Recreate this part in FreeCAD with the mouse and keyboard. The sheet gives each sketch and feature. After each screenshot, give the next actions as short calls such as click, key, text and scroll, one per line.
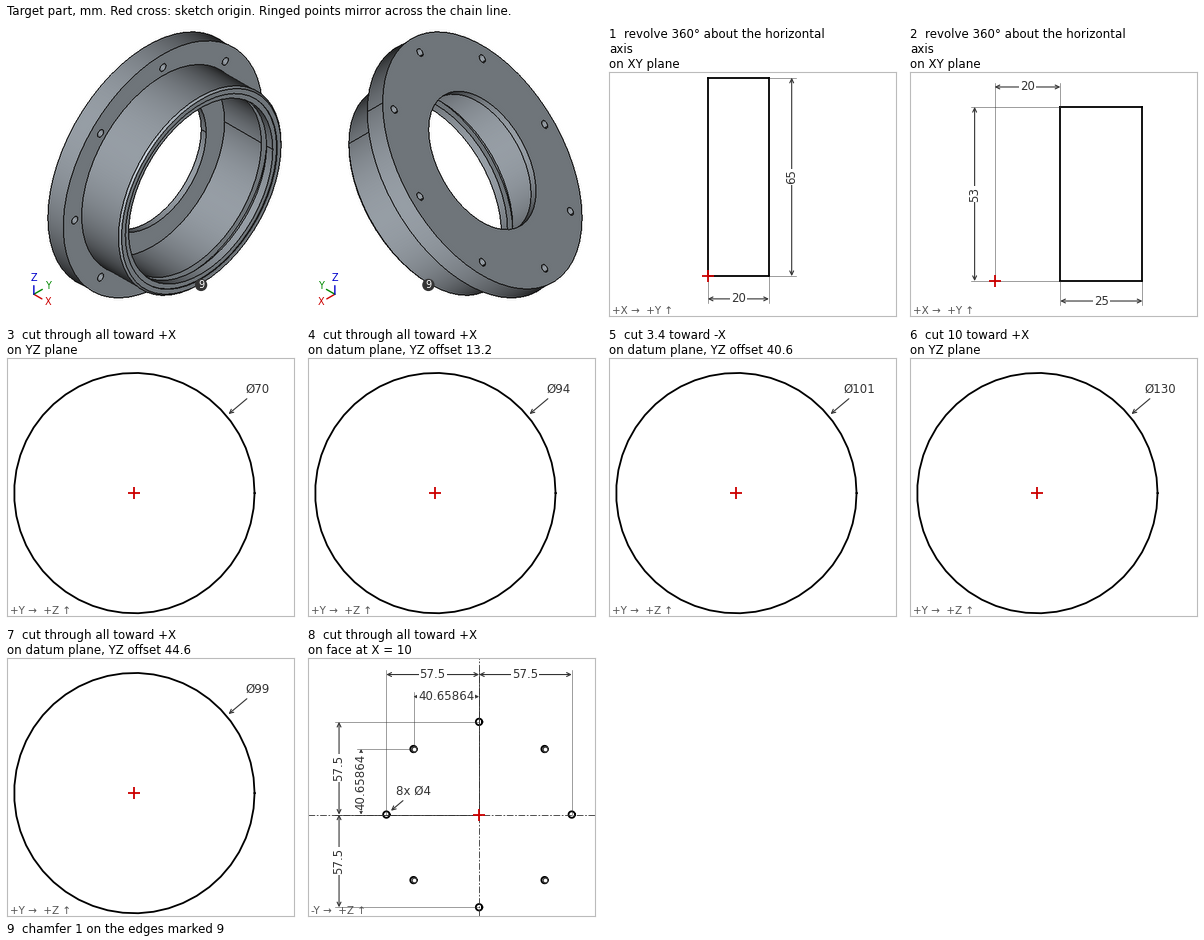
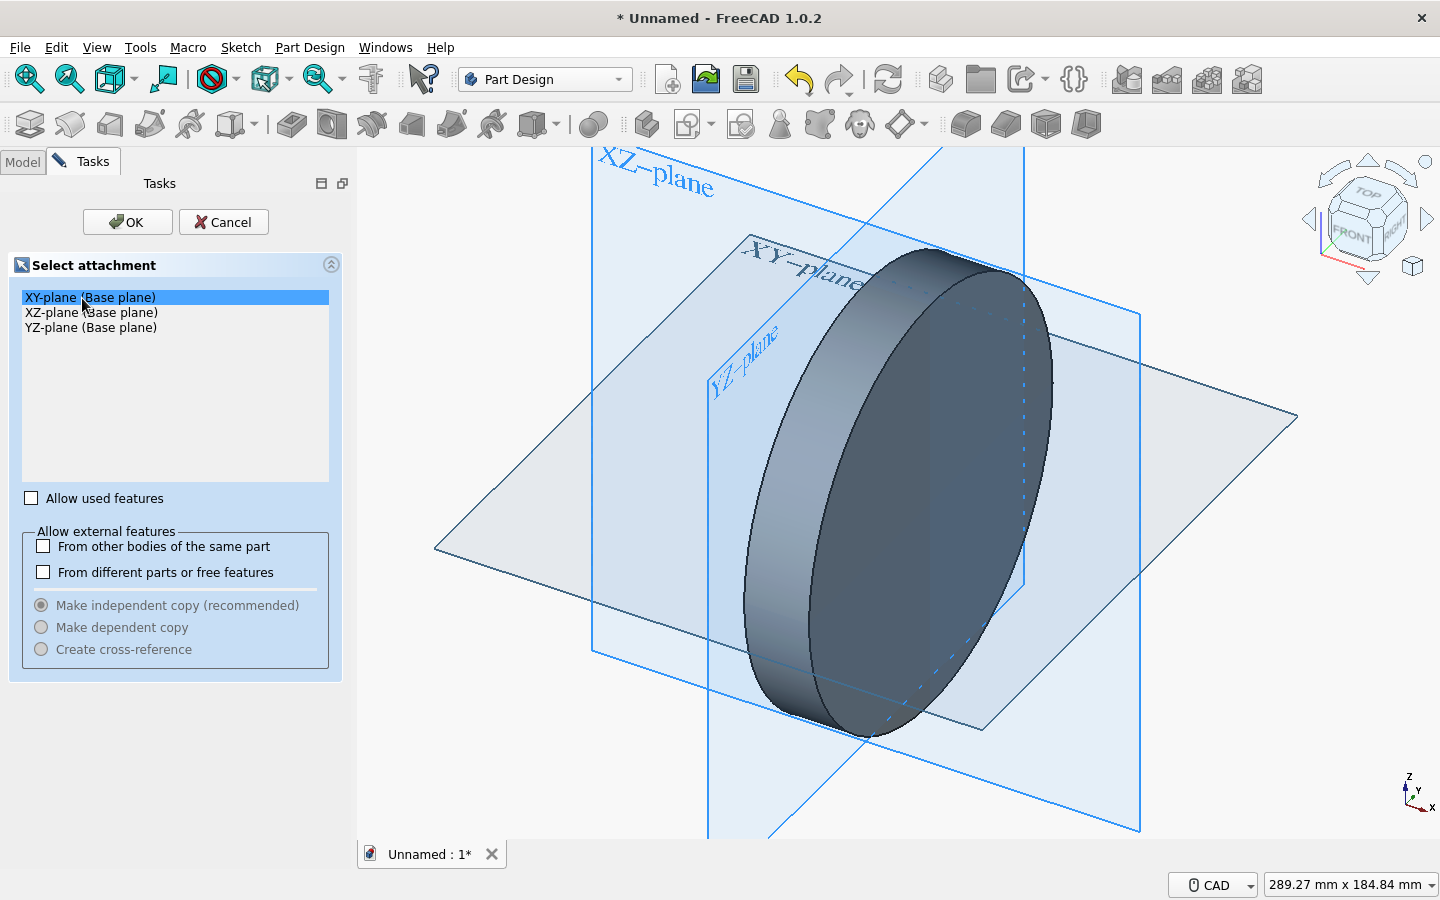
click(128, 222)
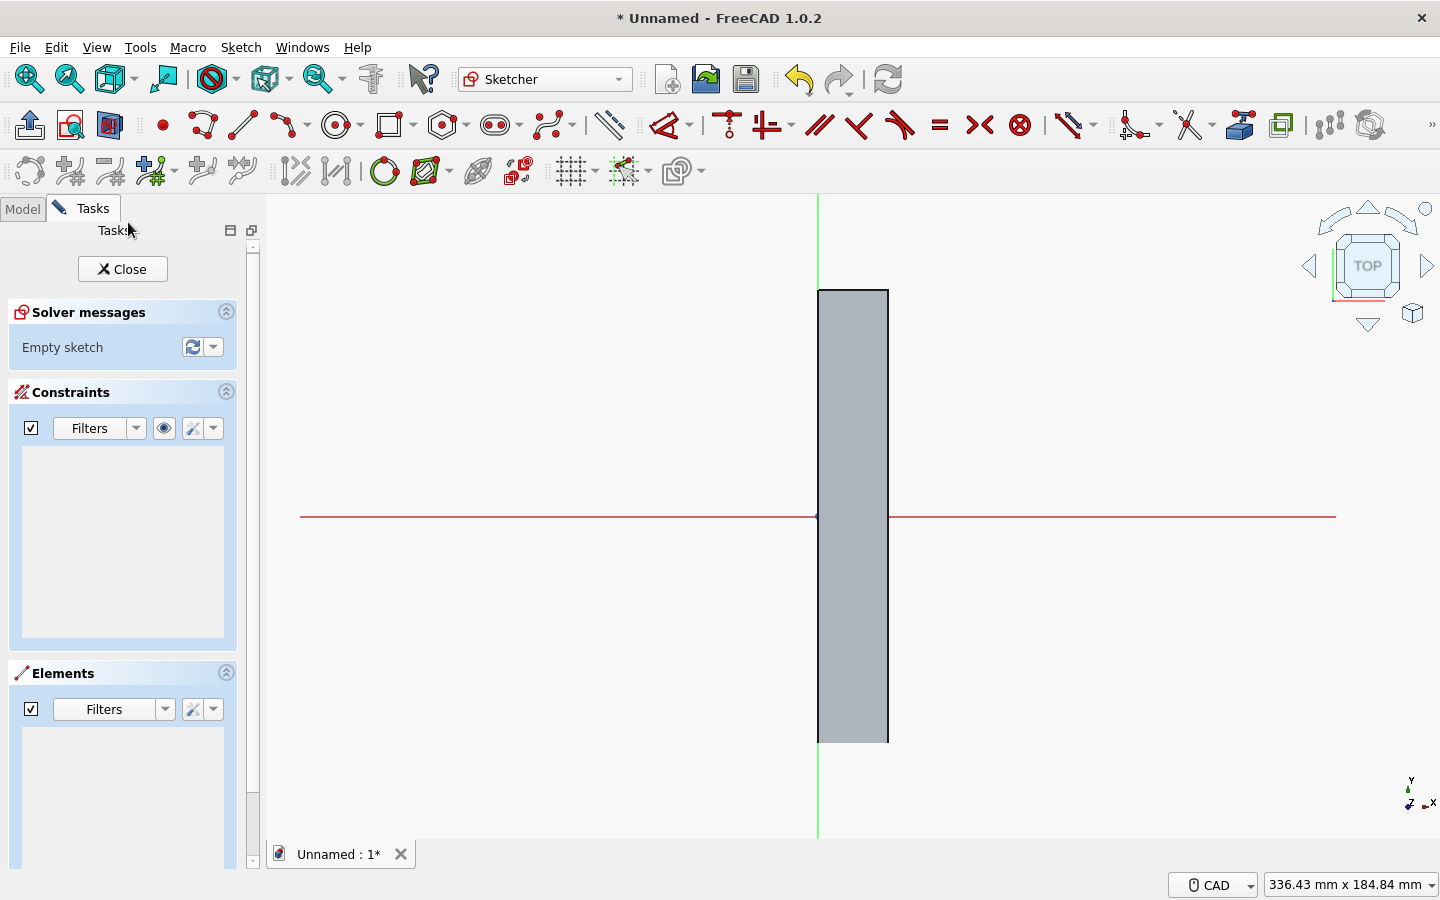
click(110, 126)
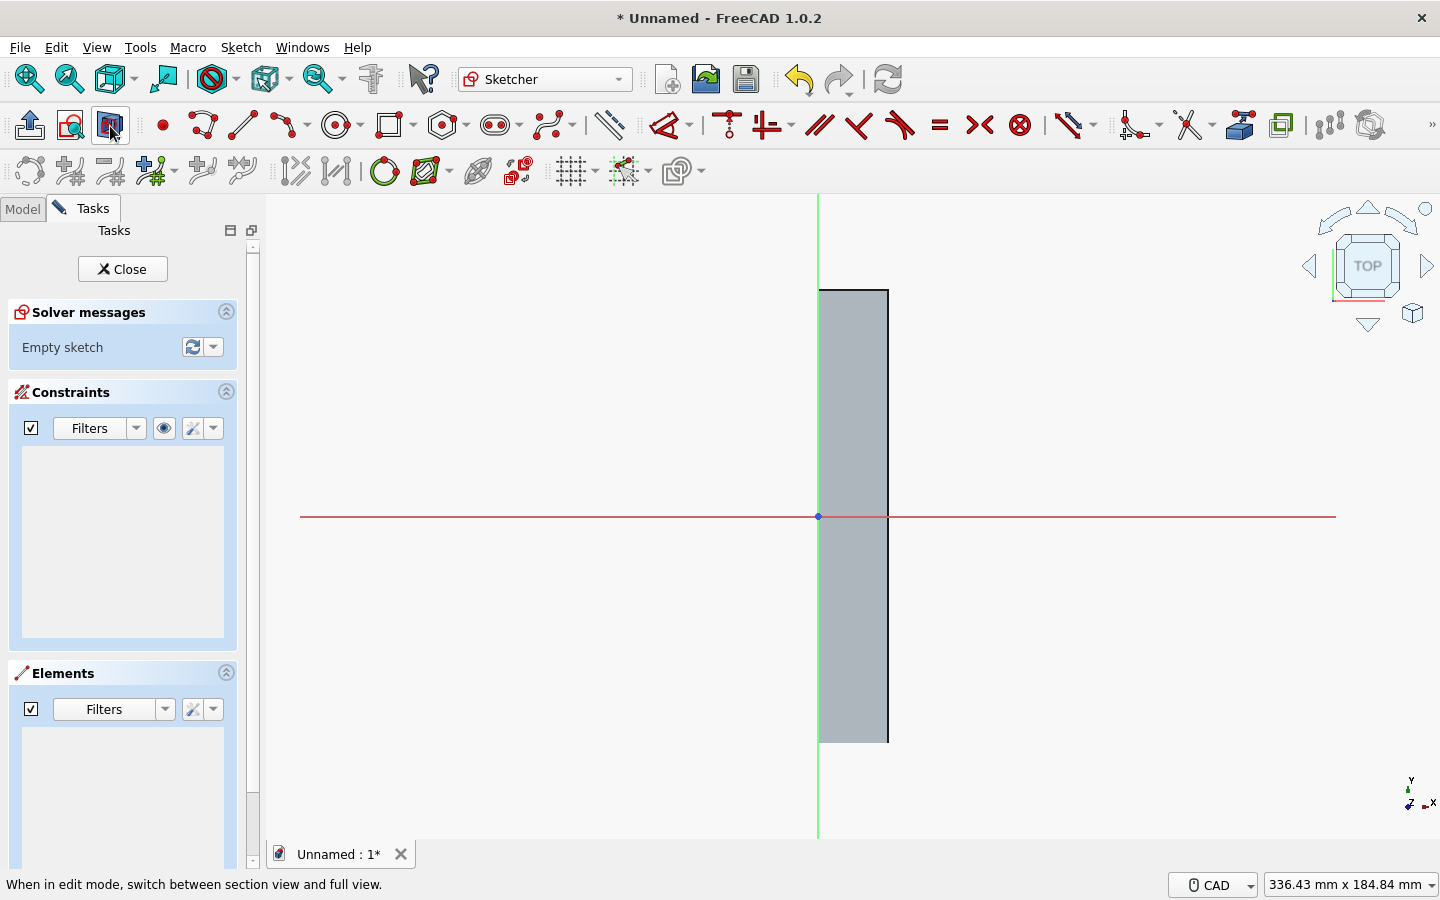
scroll(988, 349, up, 4)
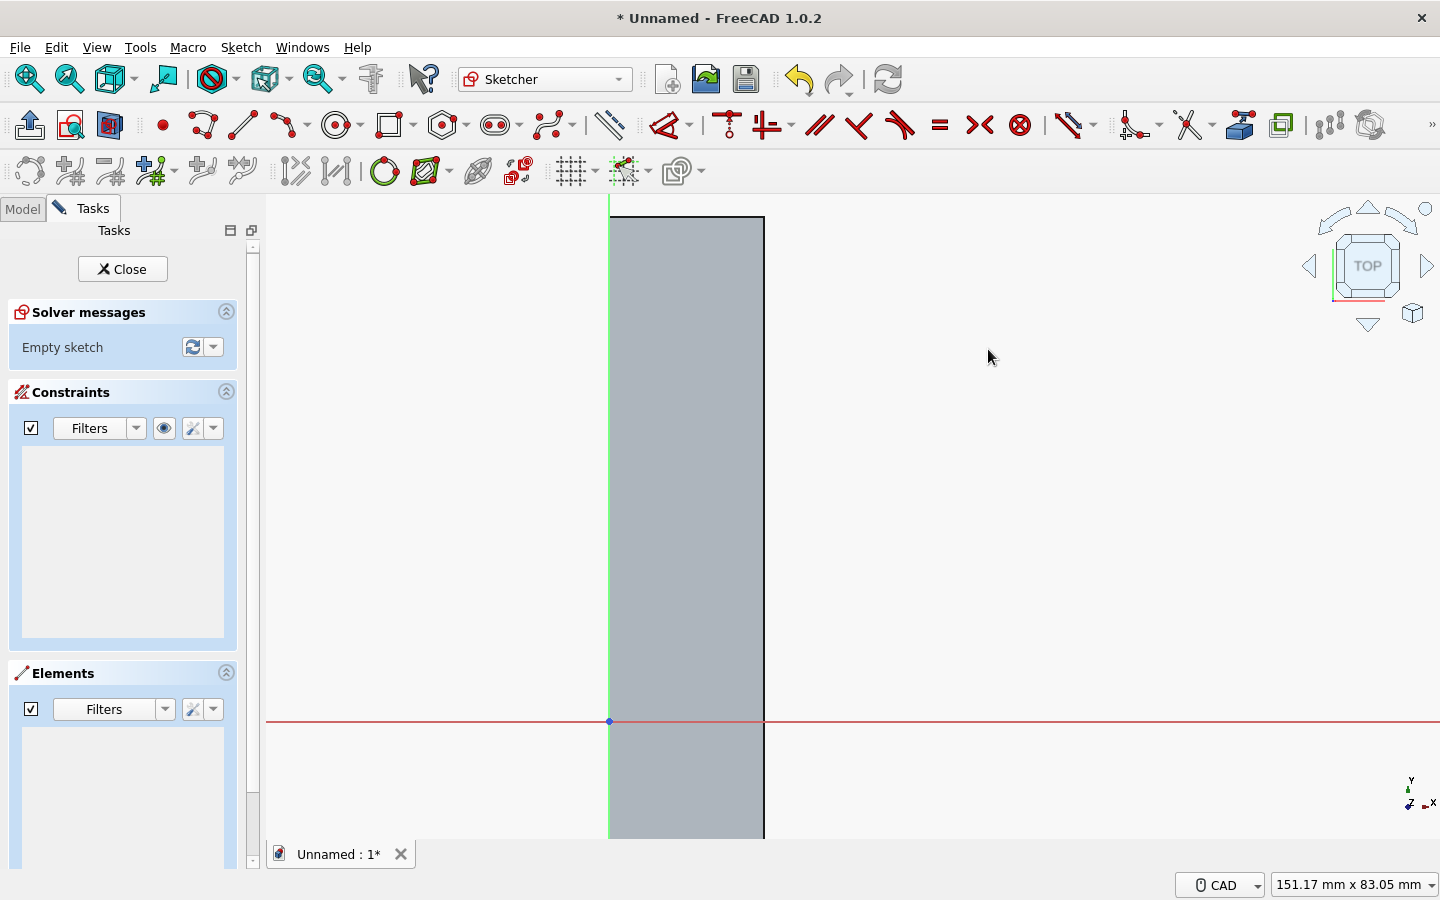
click(390, 126)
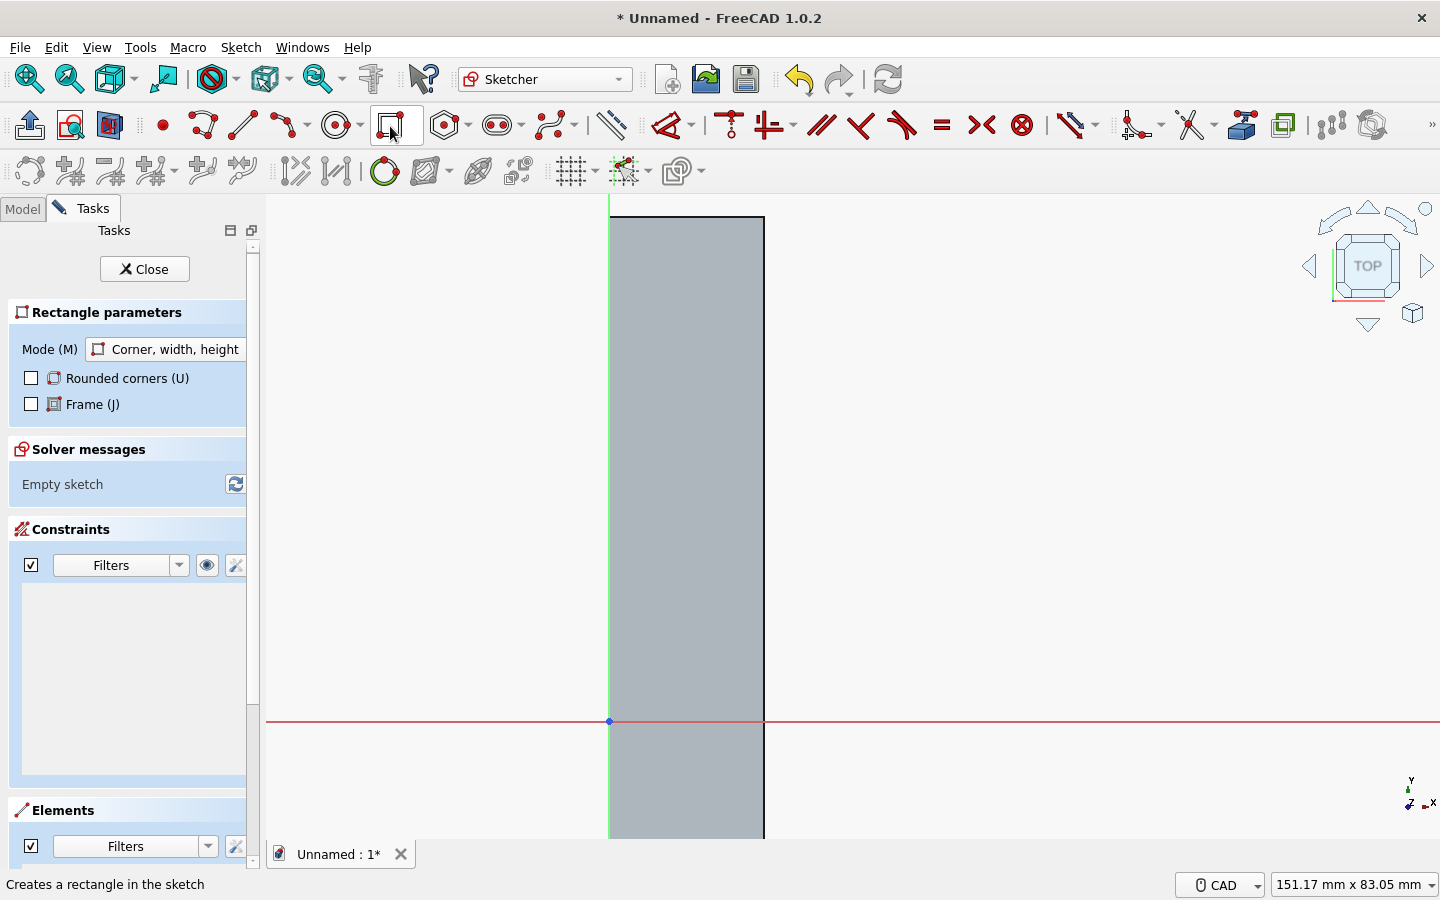
click(764, 310)
click(959, 722)
key(Escape)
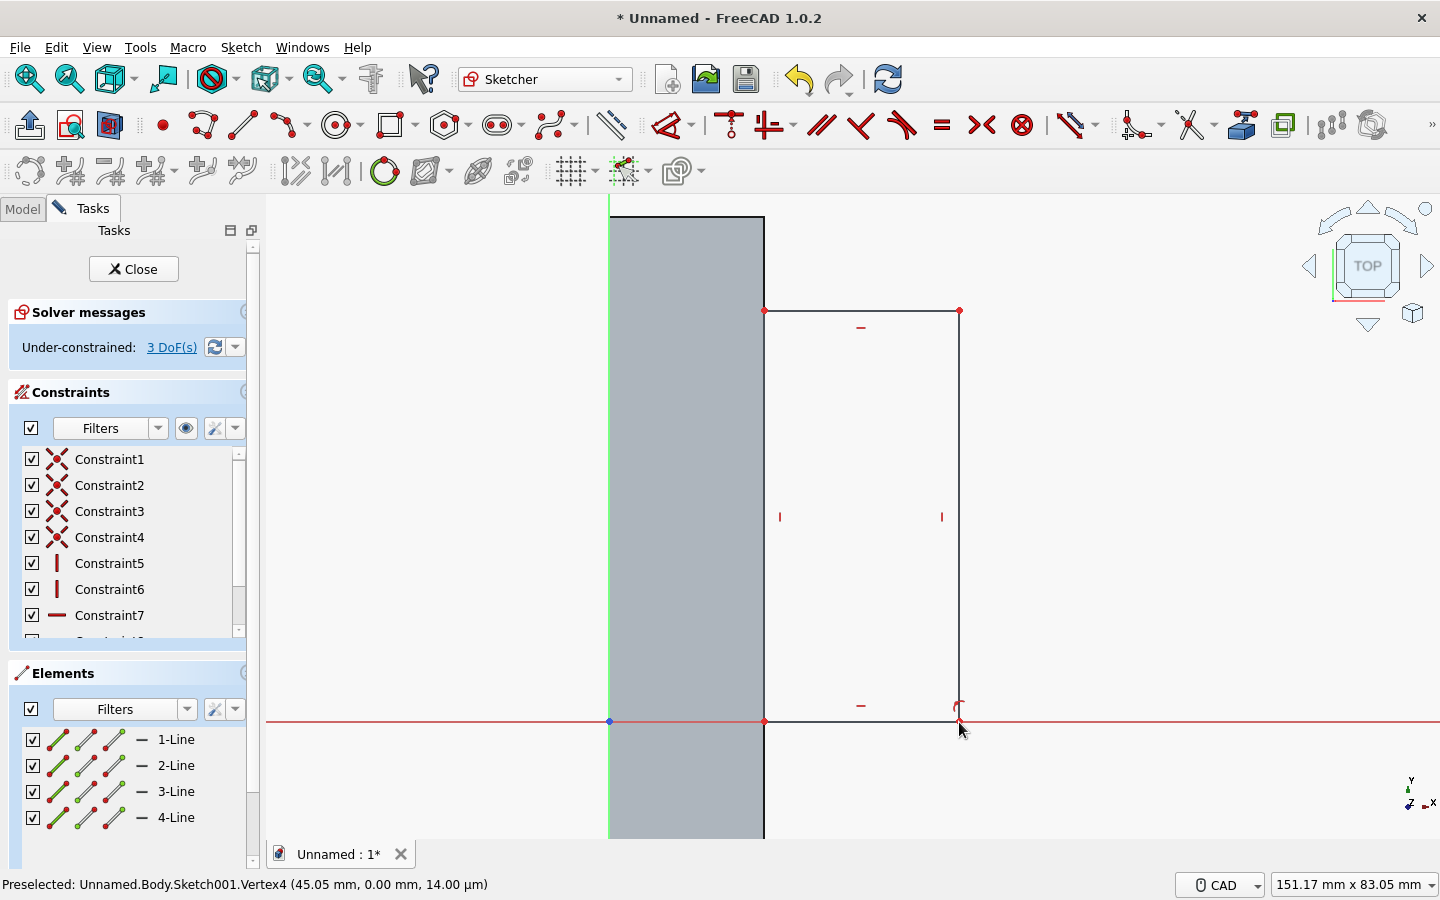
click(666, 126)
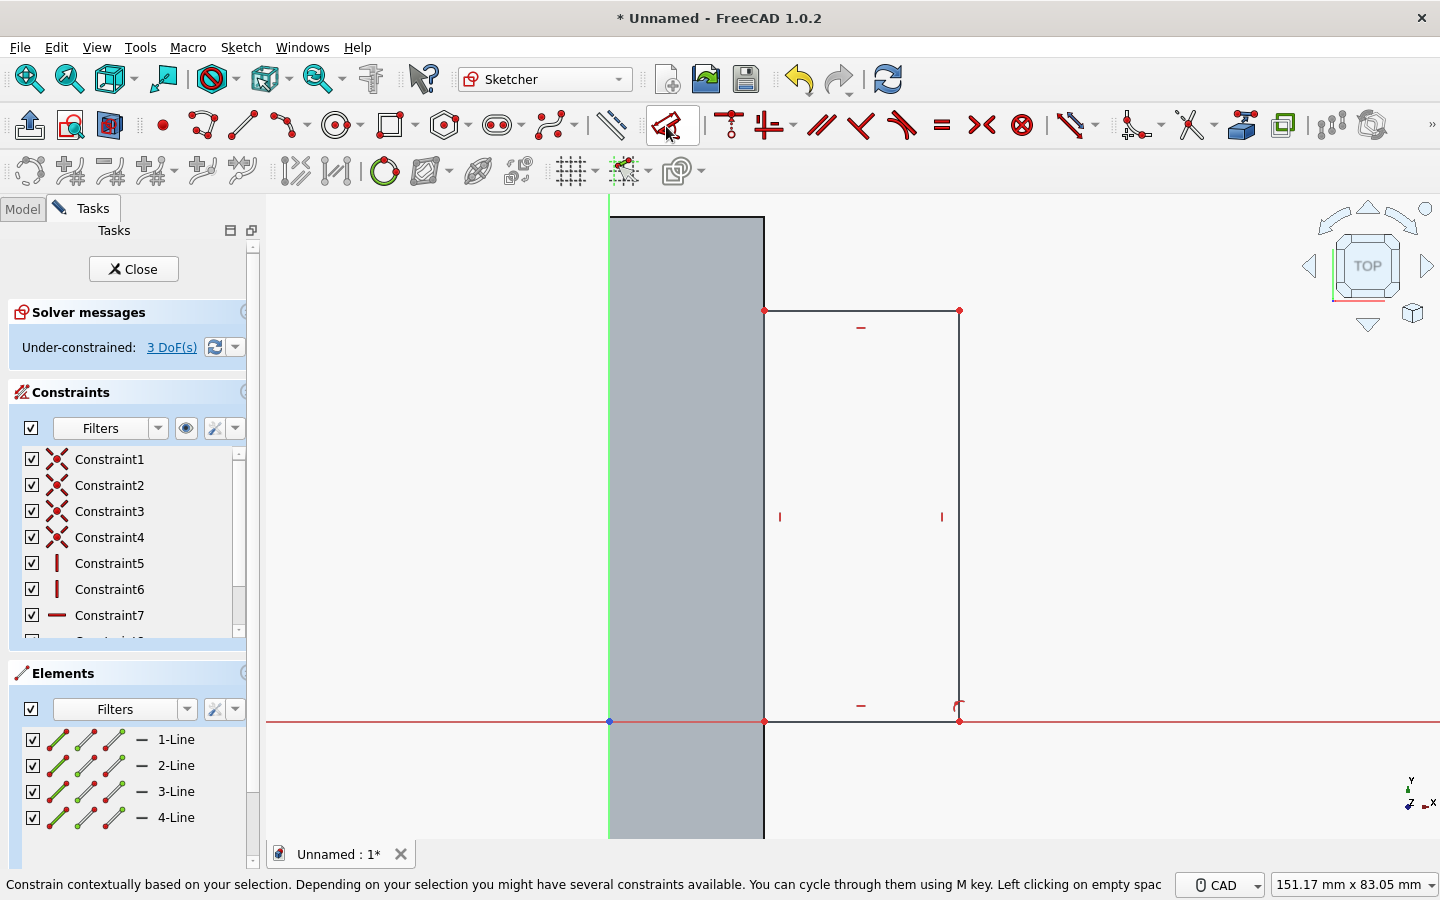
click(764, 434)
click(730, 516)